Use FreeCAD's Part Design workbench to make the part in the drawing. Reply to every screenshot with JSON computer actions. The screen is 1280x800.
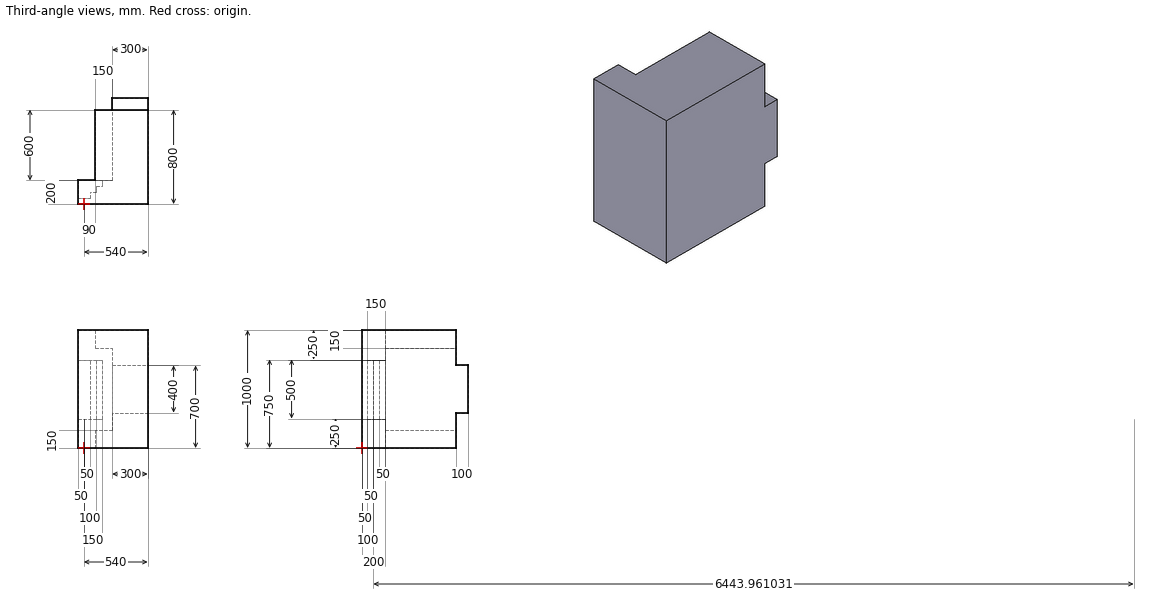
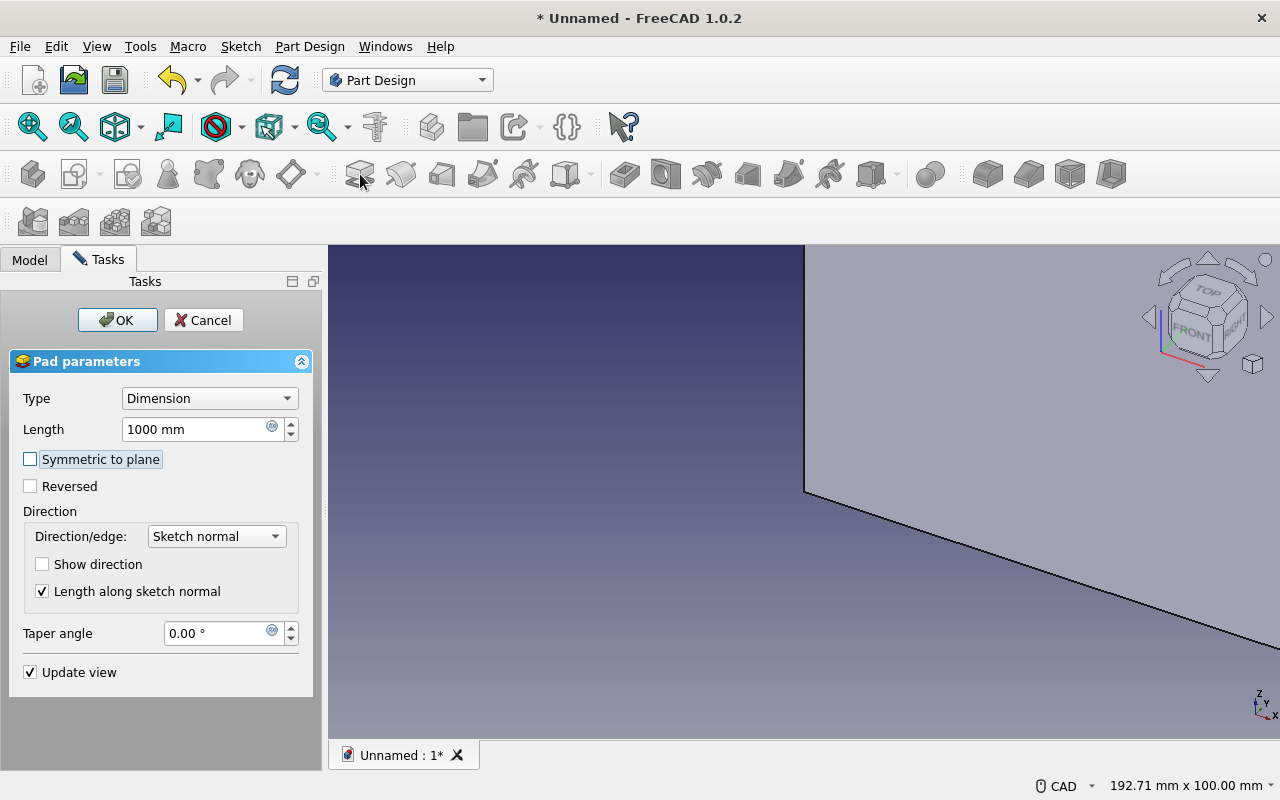
{"action": "left_click", "coordinate": [118, 320]}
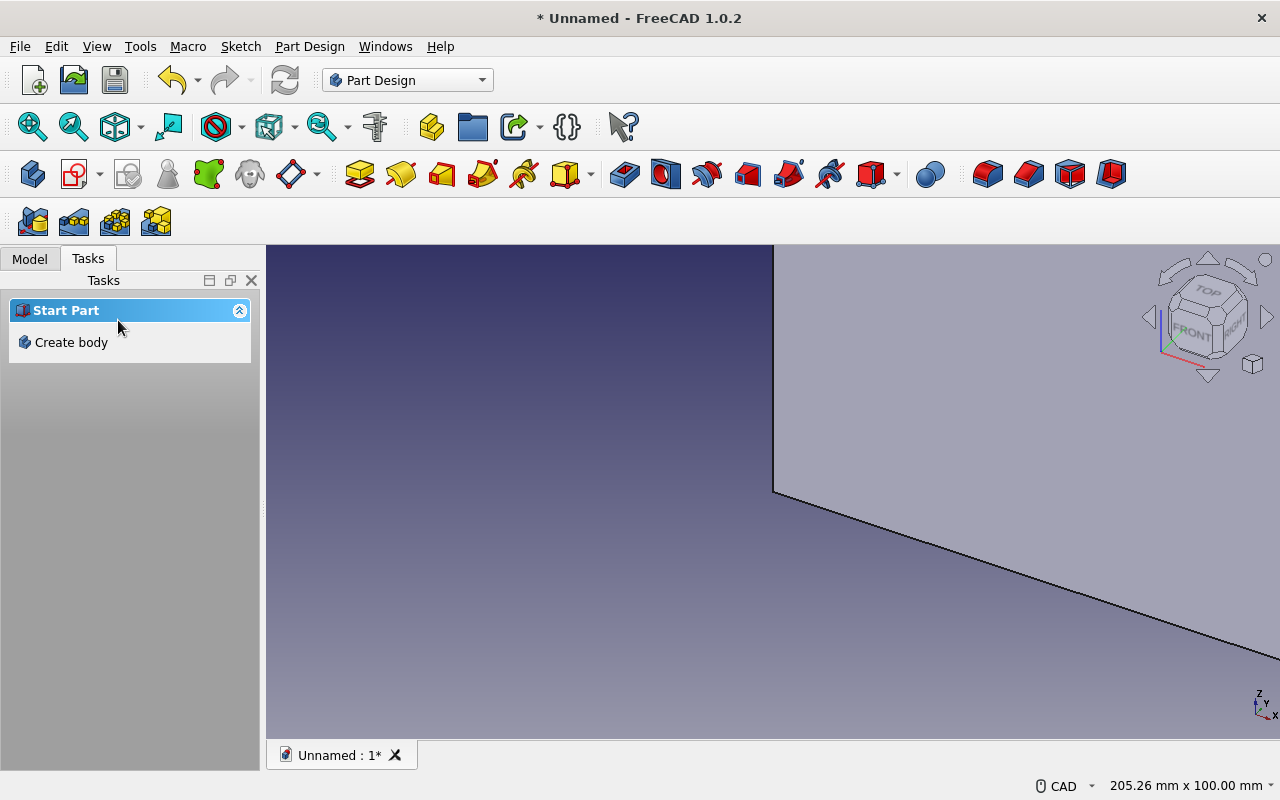
{"action": "left_click", "coordinate": [33, 128]}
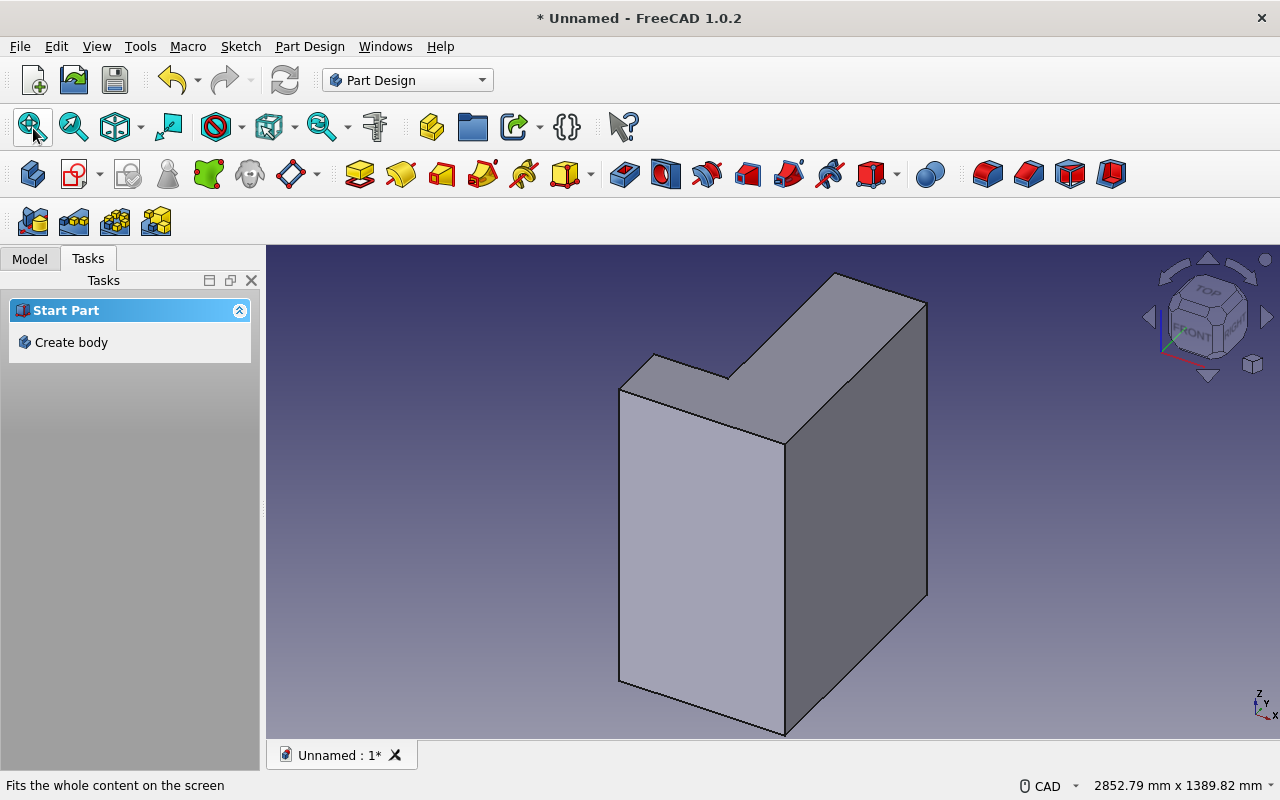
{"action": "key", "text": "5"}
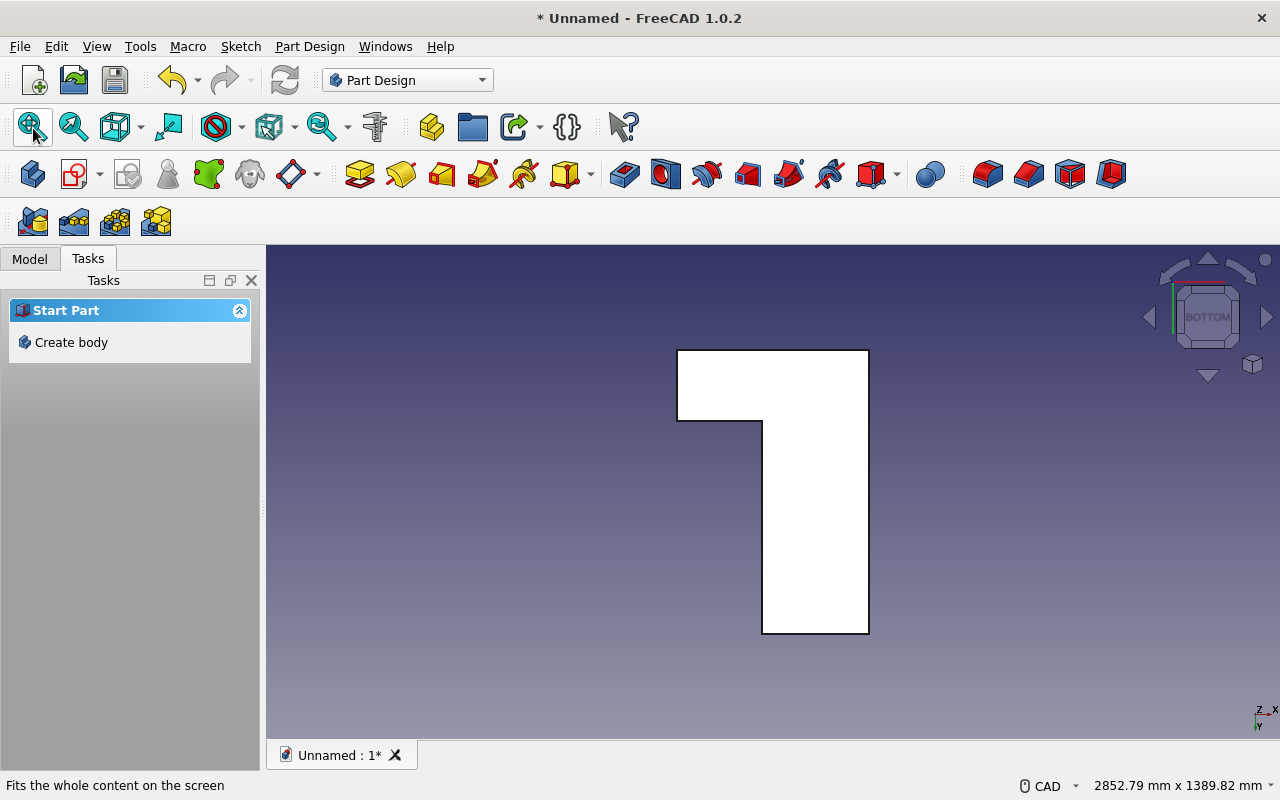
{"action": "left_click", "coordinate": [828, 572]}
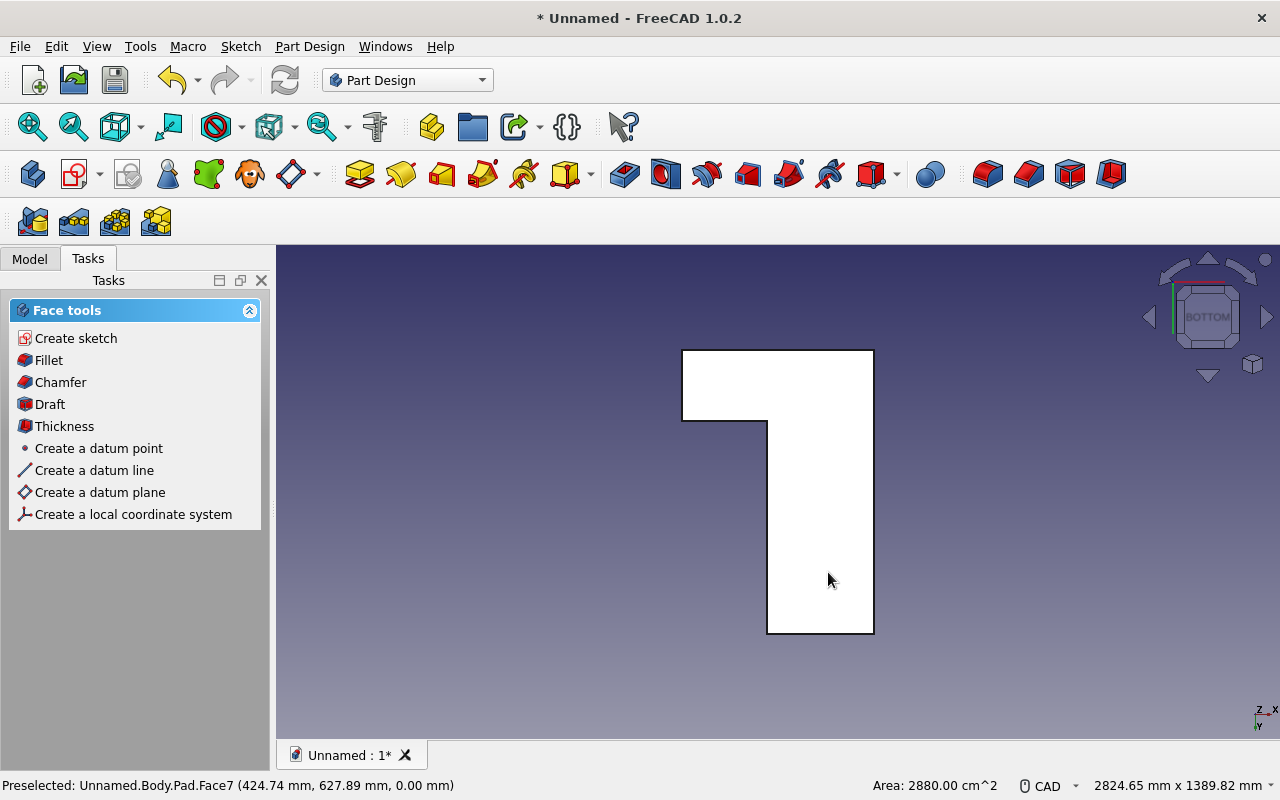
{"action": "left_click", "coordinate": [74, 174]}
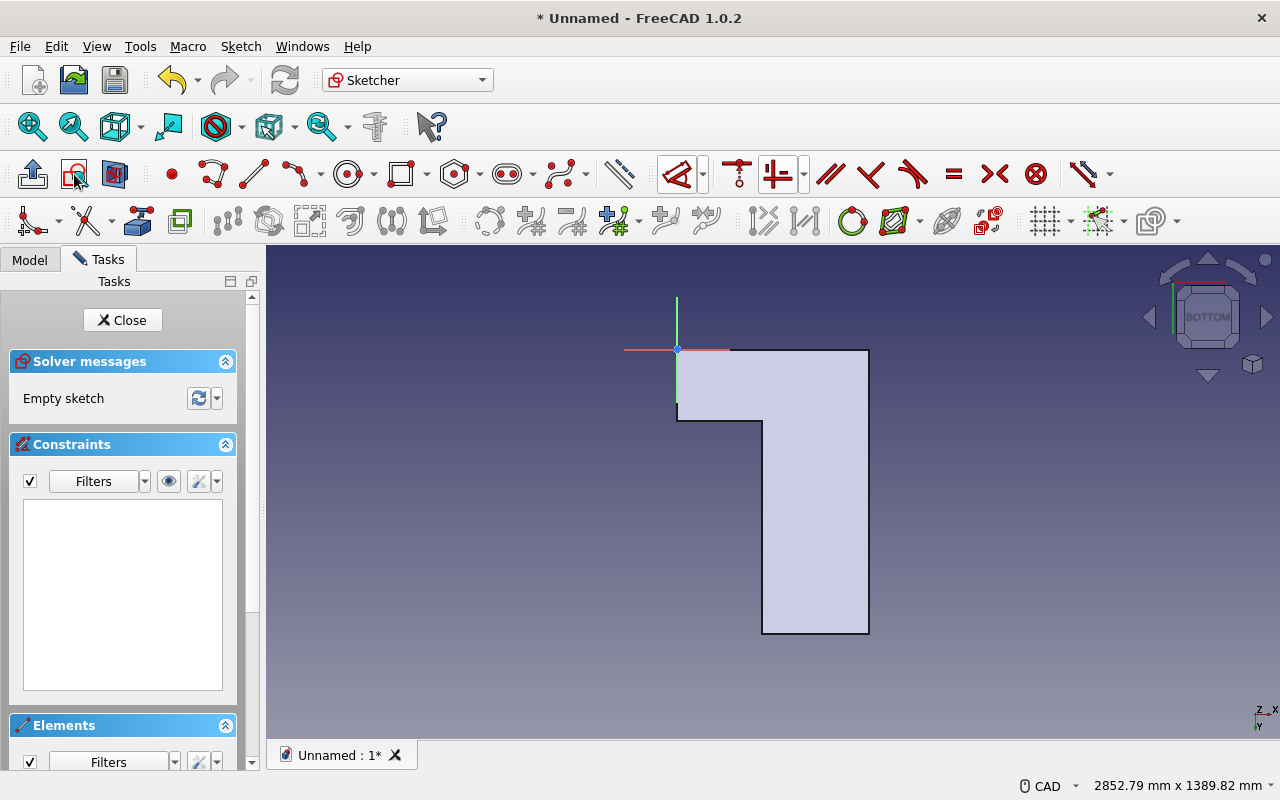
{"action": "left_click", "coordinate": [400, 174]}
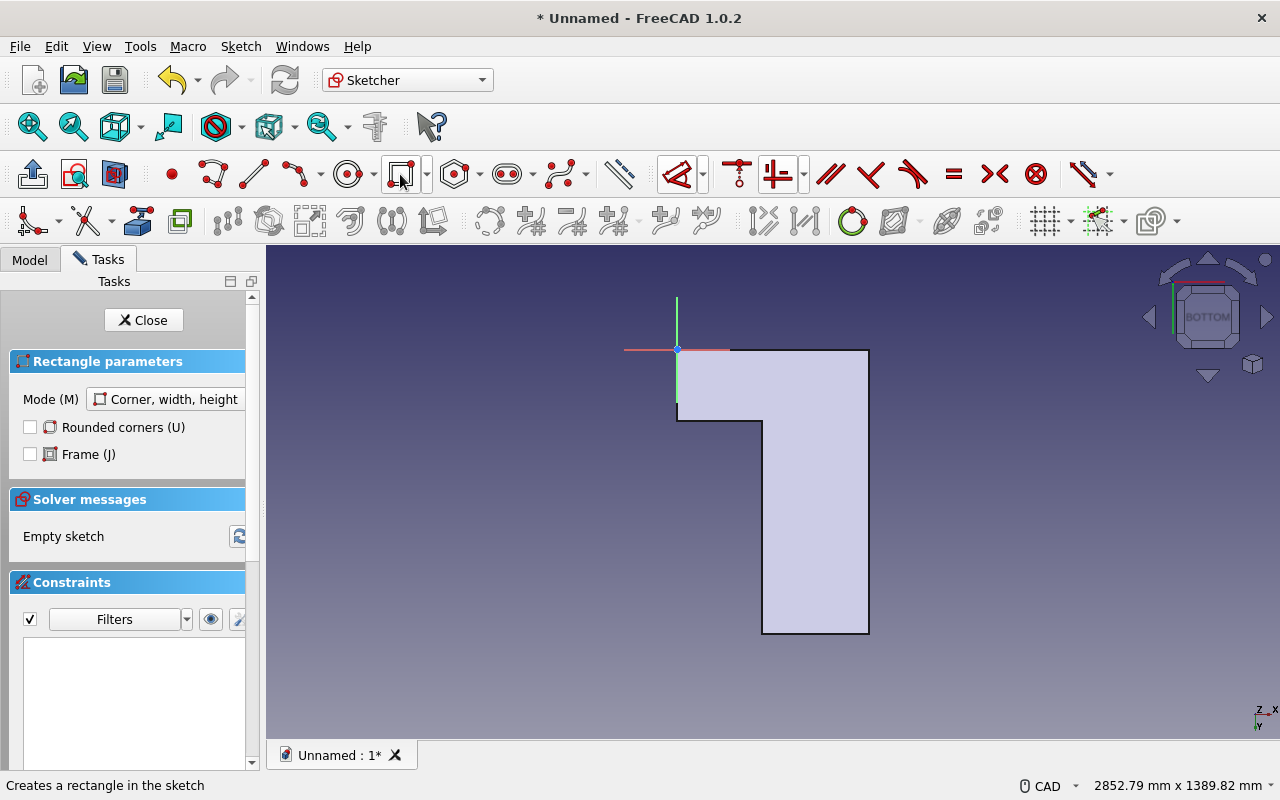
{"action": "left_click", "coordinate": [709, 421]}
{"action": "left_click", "coordinate": [762, 634]}
{"action": "key", "text": "Escape"}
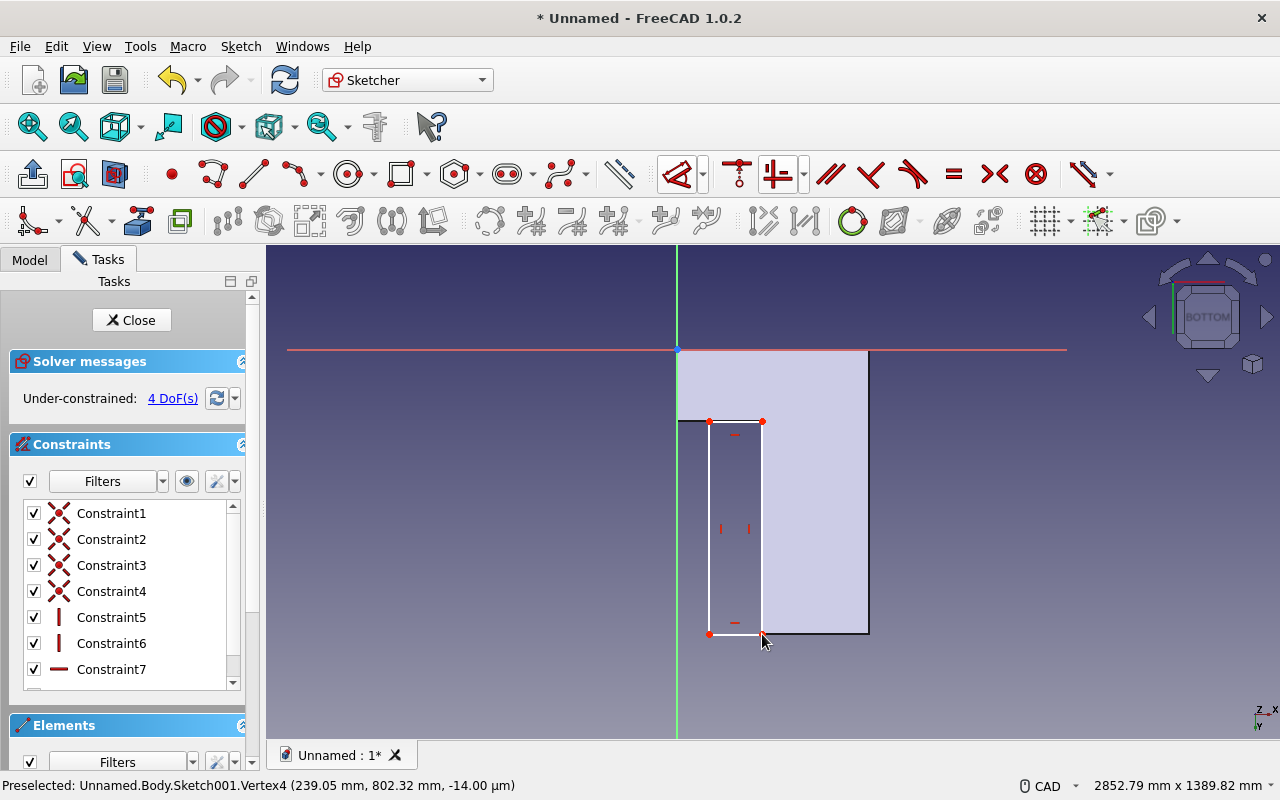
{"action": "left_click", "coordinate": [709, 486]}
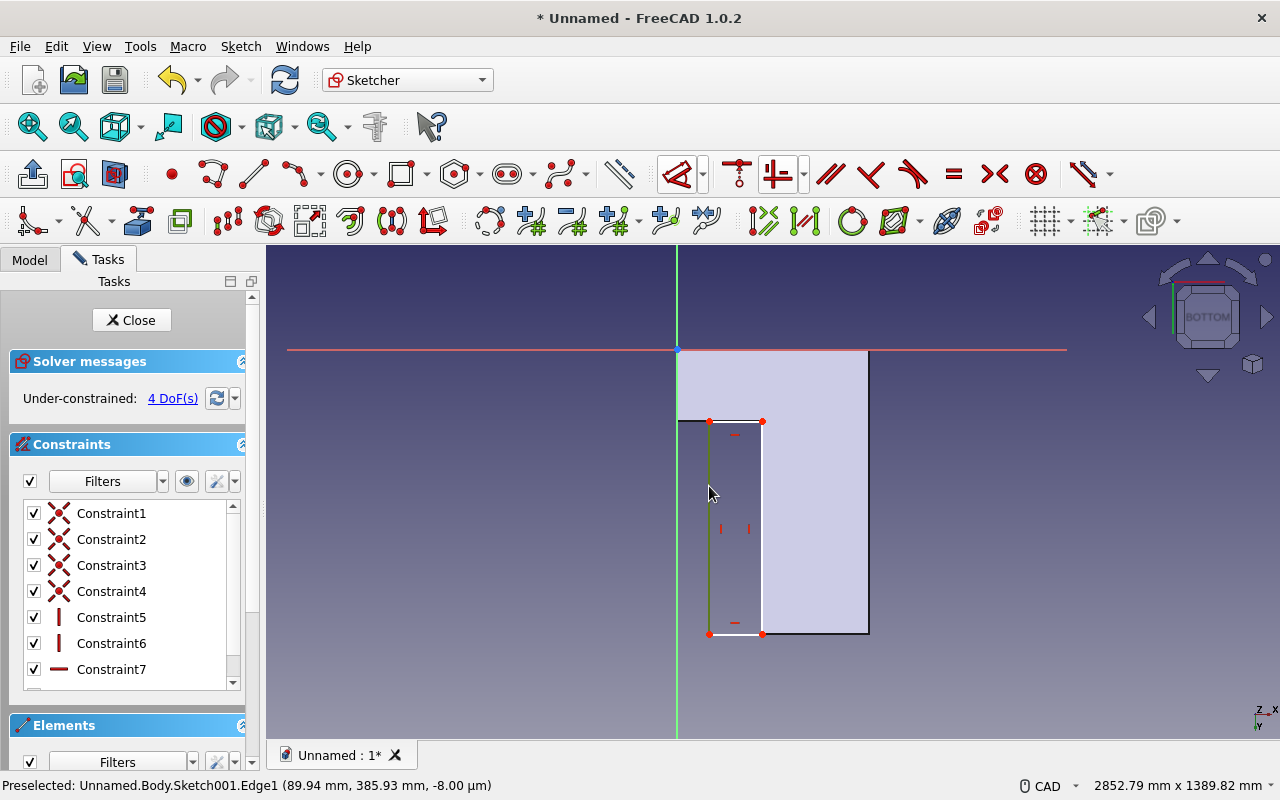
{"action": "key", "text": "i"}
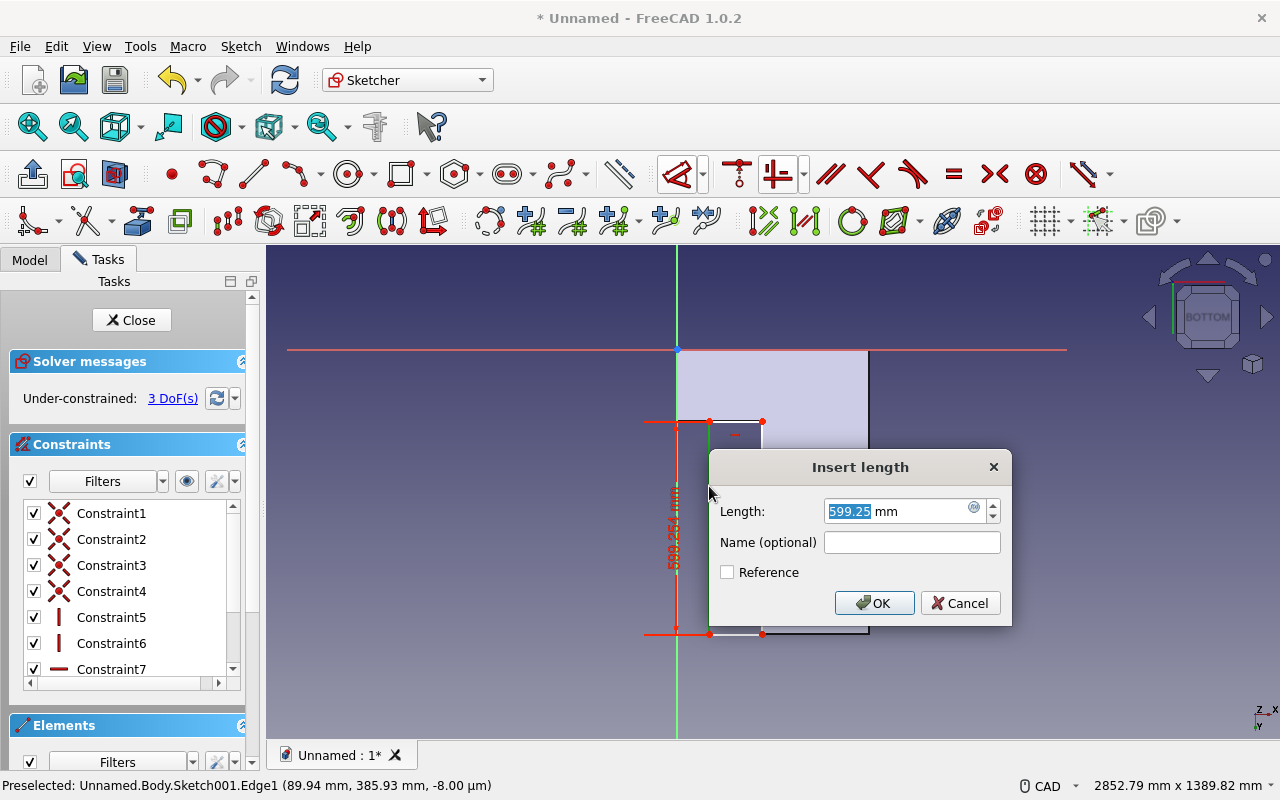
{"action": "type", "text": "600"}
{"action": "key", "text": "Return"}